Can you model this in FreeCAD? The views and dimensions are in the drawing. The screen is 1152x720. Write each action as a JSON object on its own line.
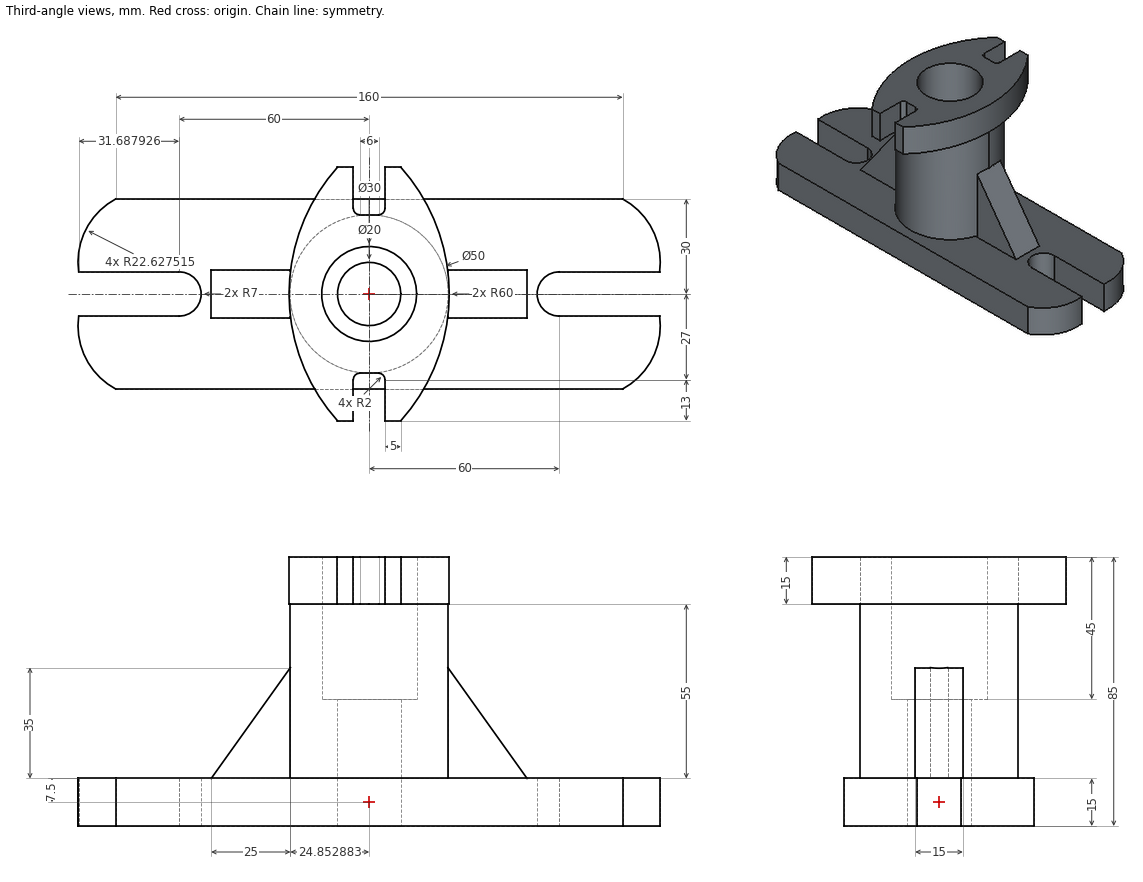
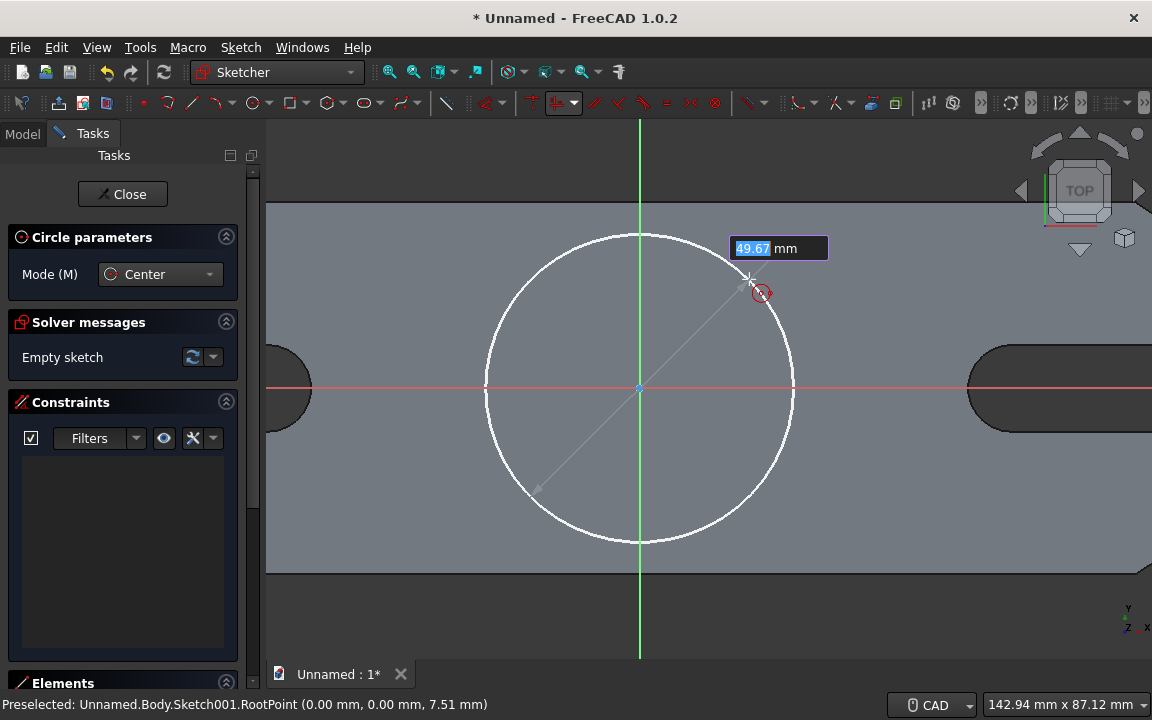
{"action": "type", "text": "50"}
{"action": "key", "text": "Return"}
{"action": "key", "text": "Escape"}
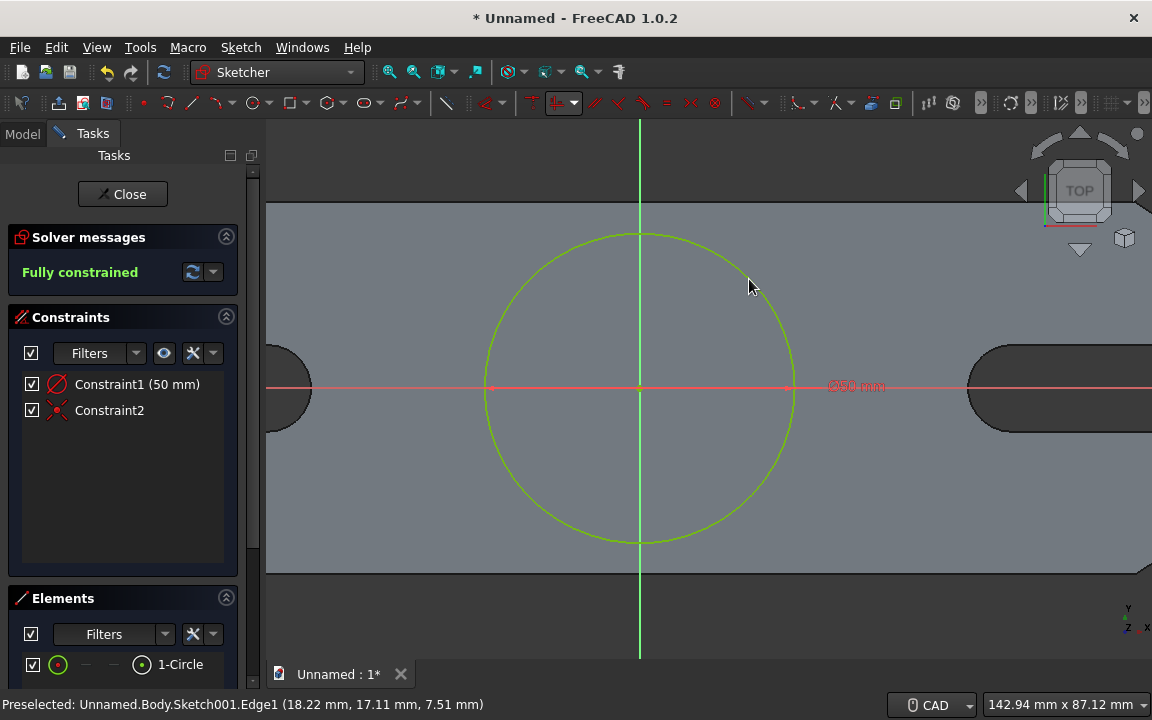
{"action": "left_click", "coordinate": [123, 194]}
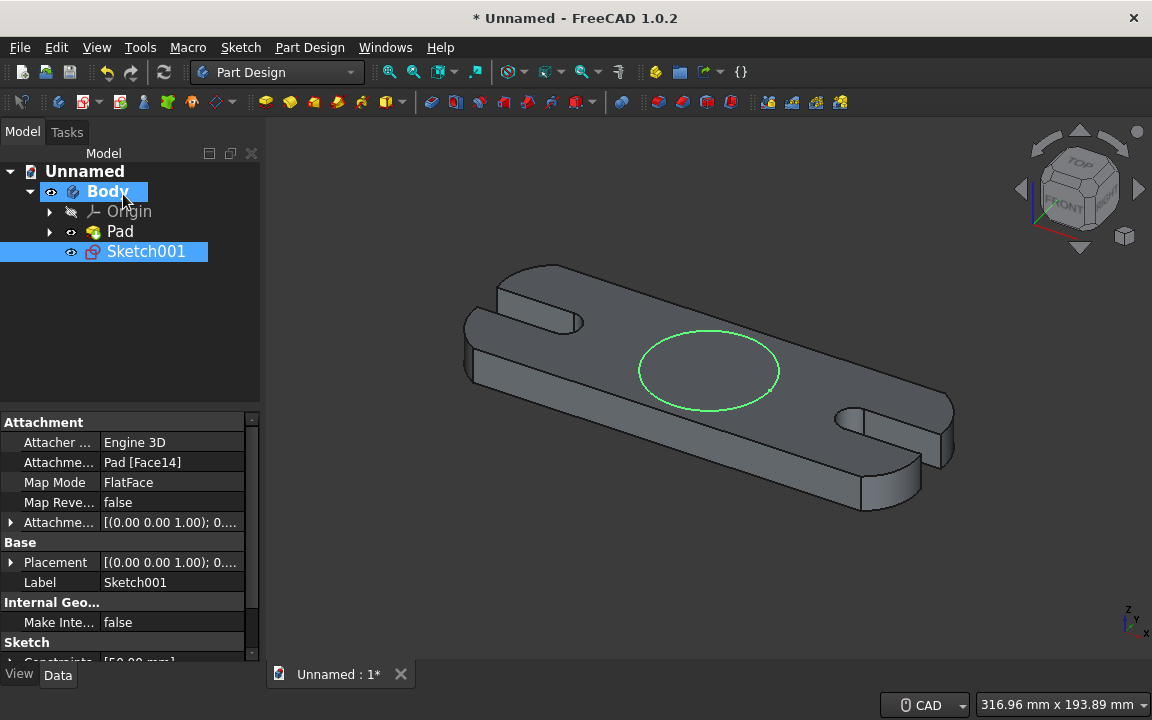
{"action": "left_click", "coordinate": [266, 102]}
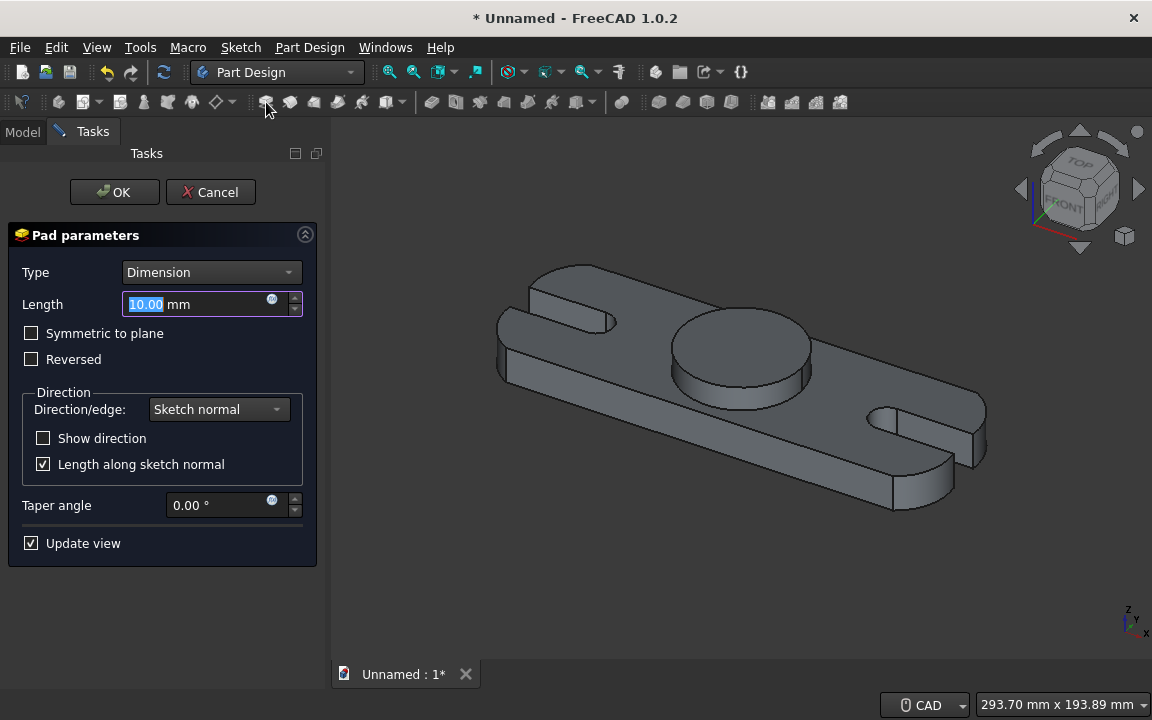
{"action": "type", "text": "55"}
{"action": "key", "text": "Tab"}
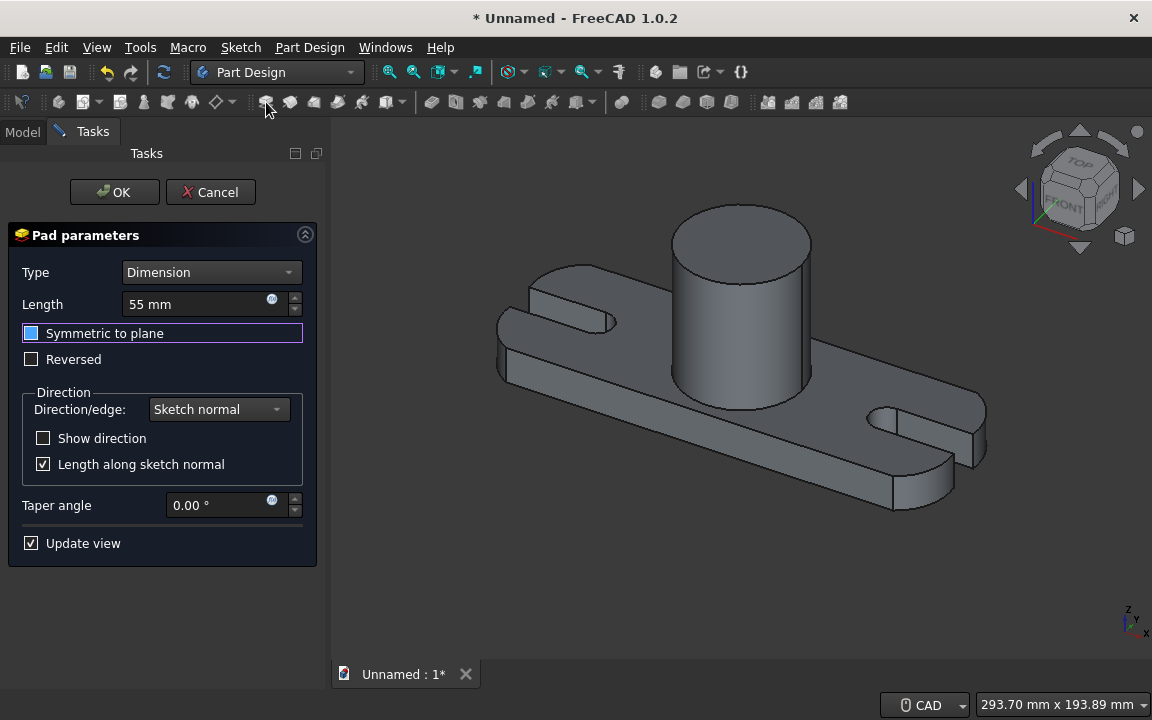
{"action": "left_click", "coordinate": [115, 192]}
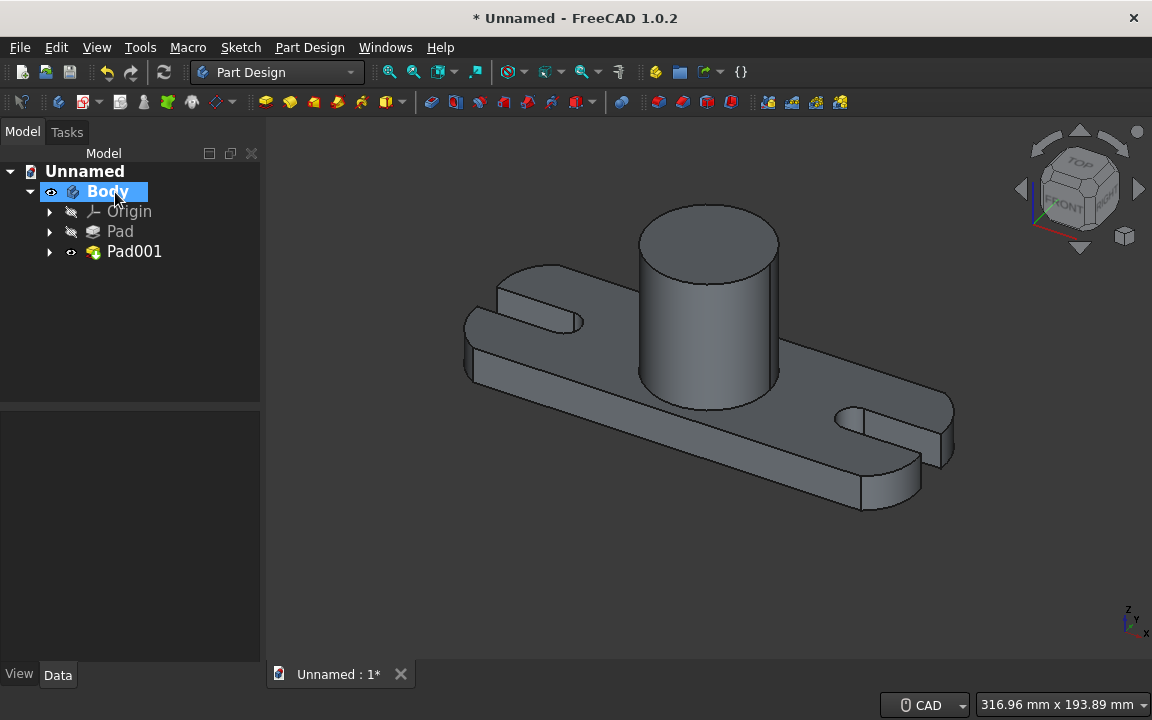
{"action": "left_click", "coordinate": [709, 243]}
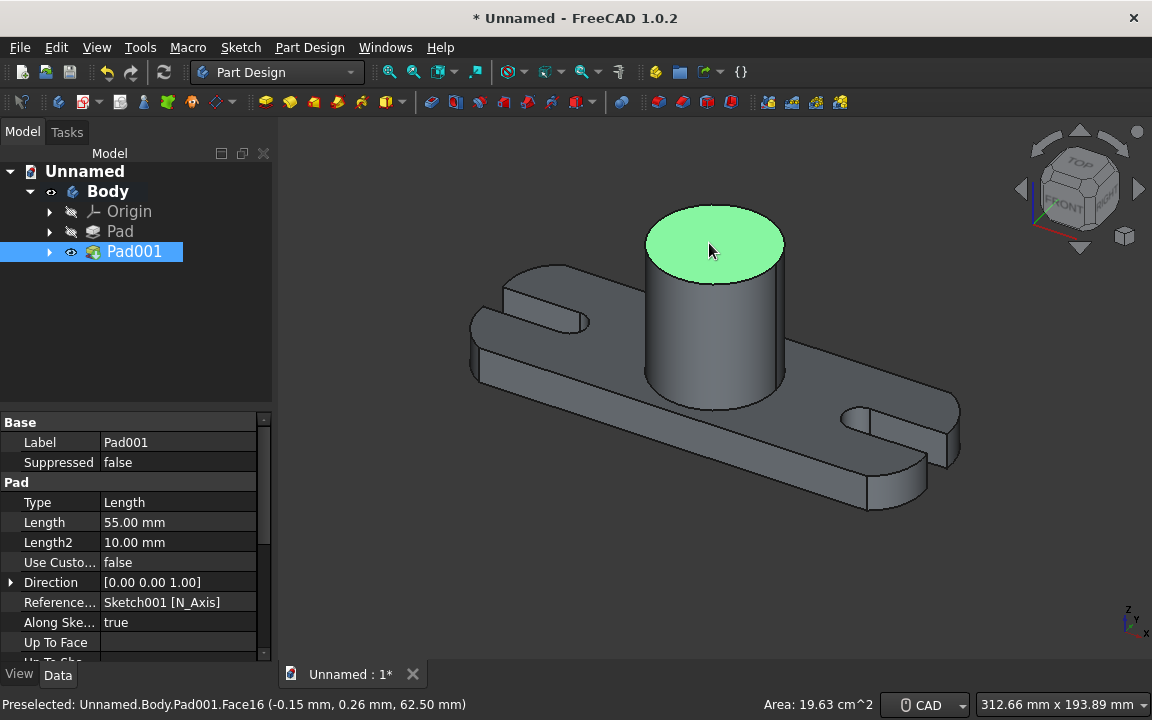
{"action": "left_click", "coordinate": [84, 102]}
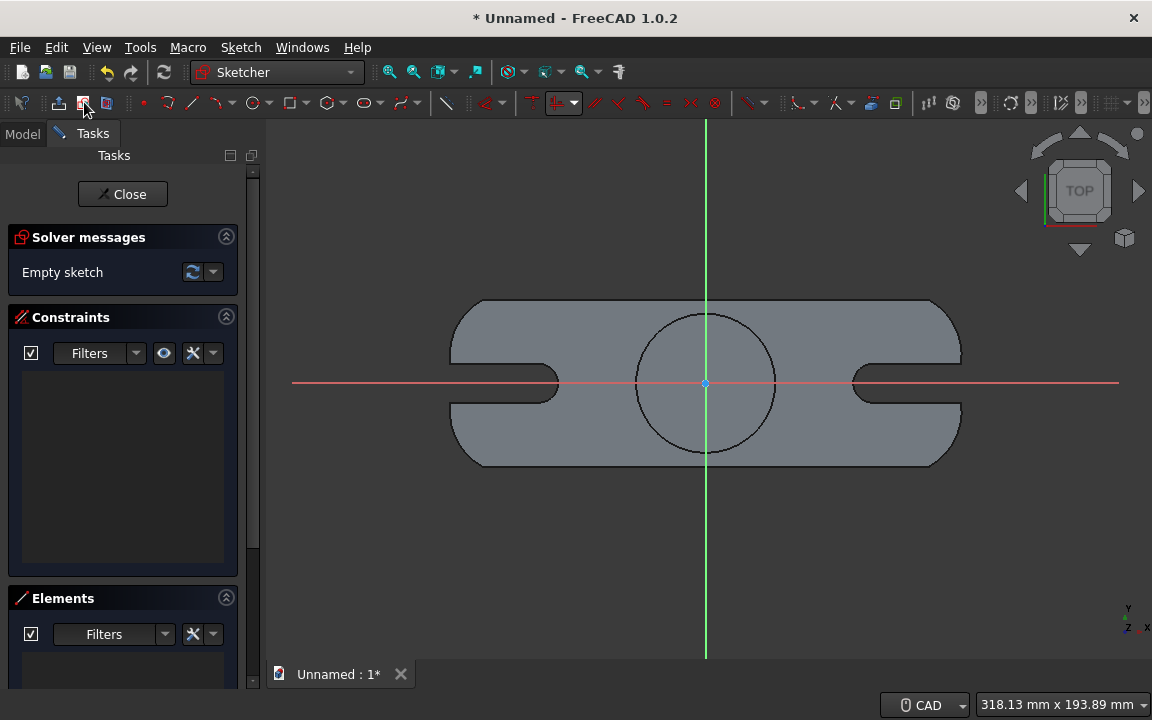
{"action": "scroll", "coordinate": [727, 381], "scroll_direction": "up", "scroll_amount": 7}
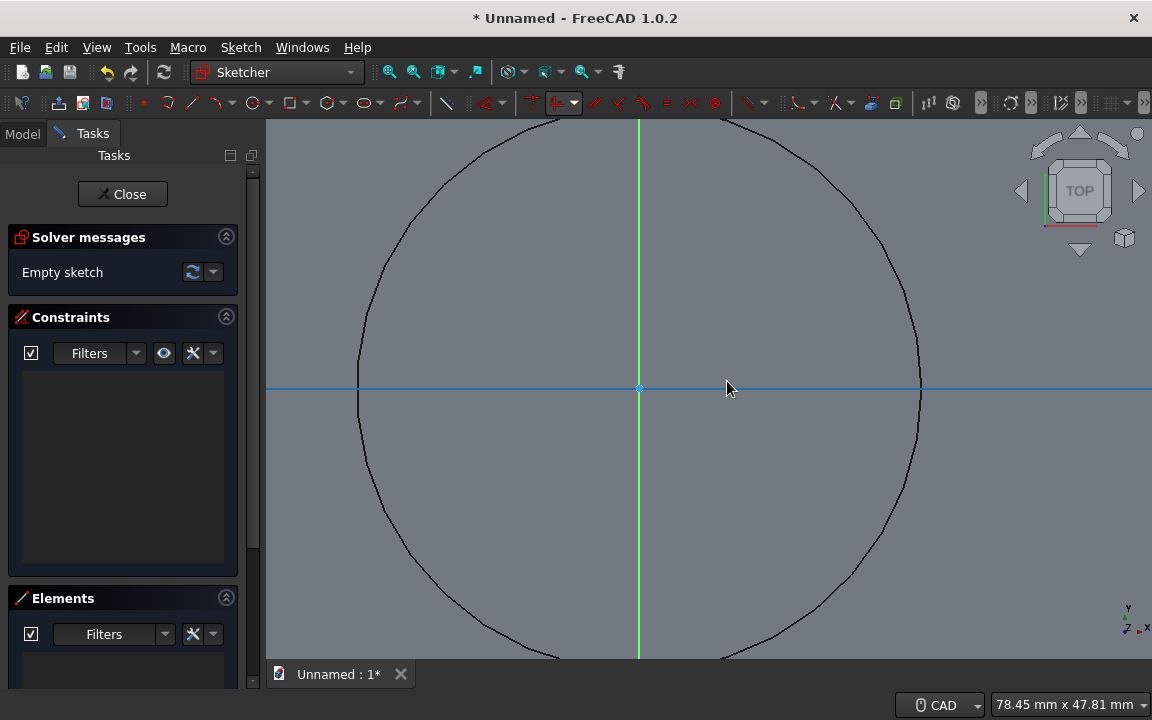
{"action": "left_click", "coordinate": [254, 104]}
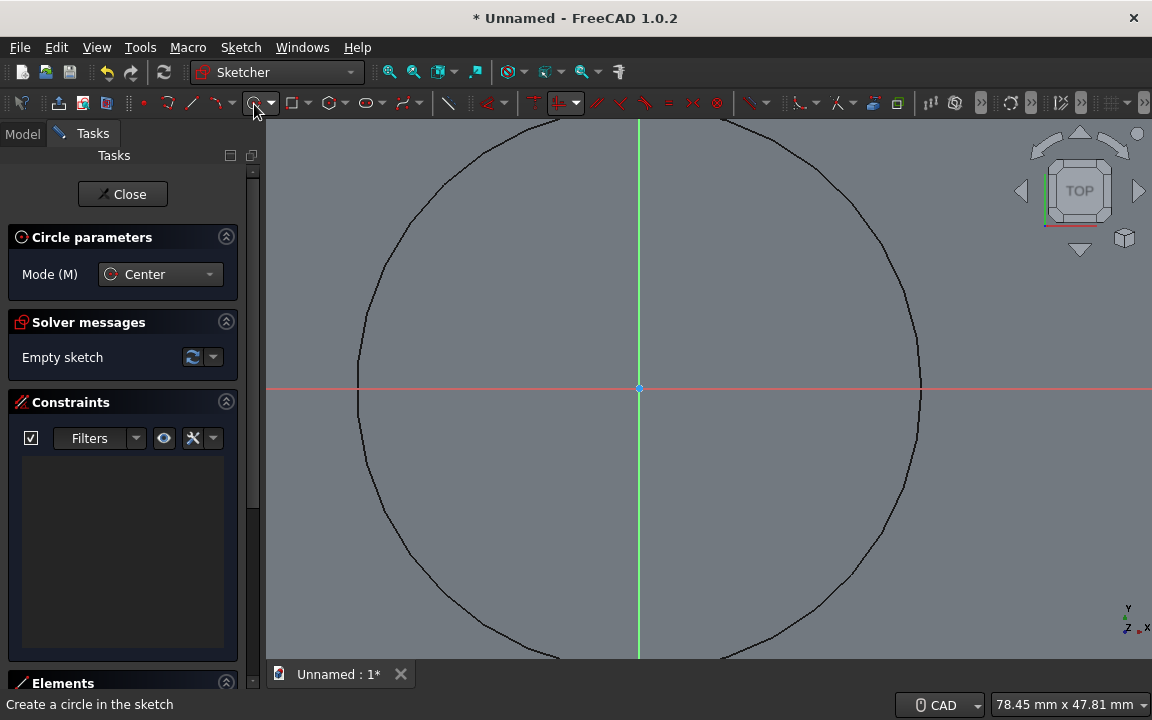
{"action": "left_click", "coordinate": [639, 389]}
{"action": "mouse_move", "coordinate": [759, 269]}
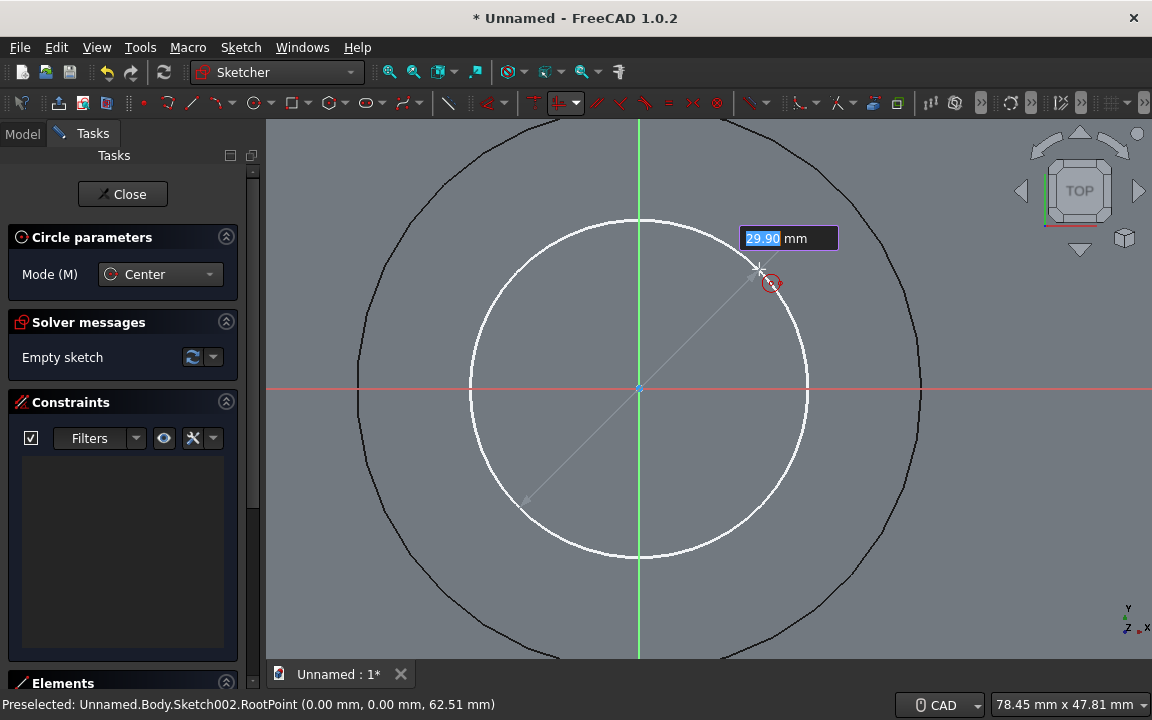
{"action": "type", "text": "30"}
{"action": "key", "text": "Return"}
{"action": "key", "text": "Escape"}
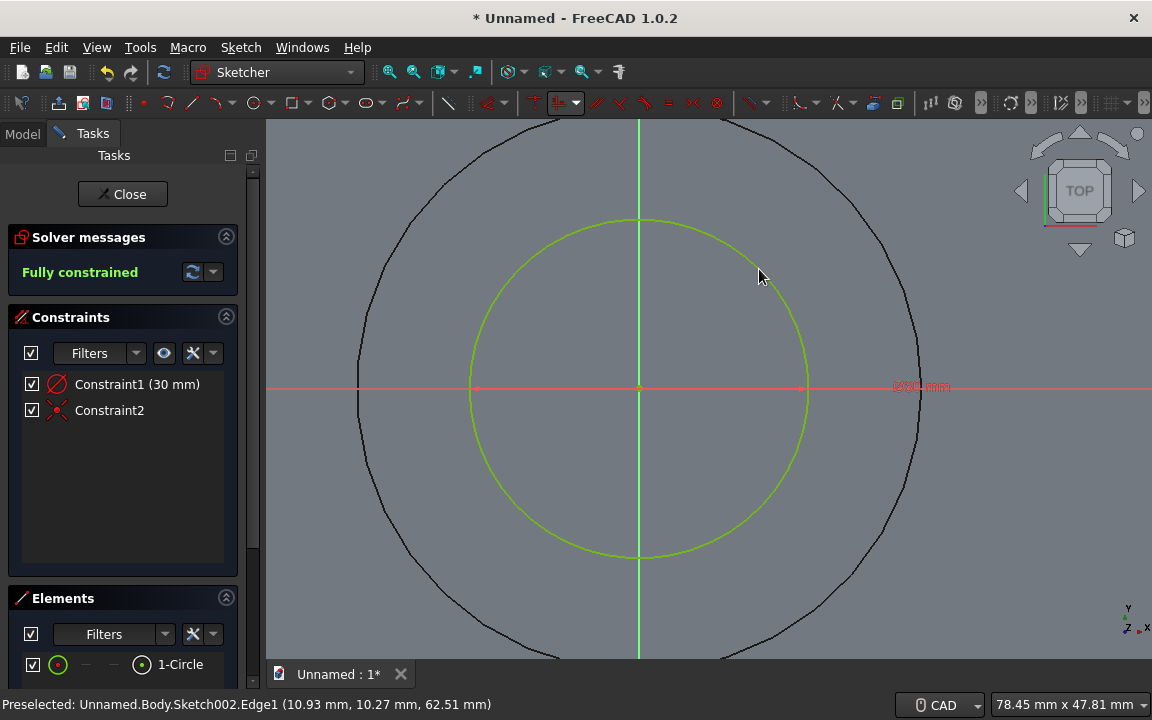
{"action": "left_click", "coordinate": [123, 194]}